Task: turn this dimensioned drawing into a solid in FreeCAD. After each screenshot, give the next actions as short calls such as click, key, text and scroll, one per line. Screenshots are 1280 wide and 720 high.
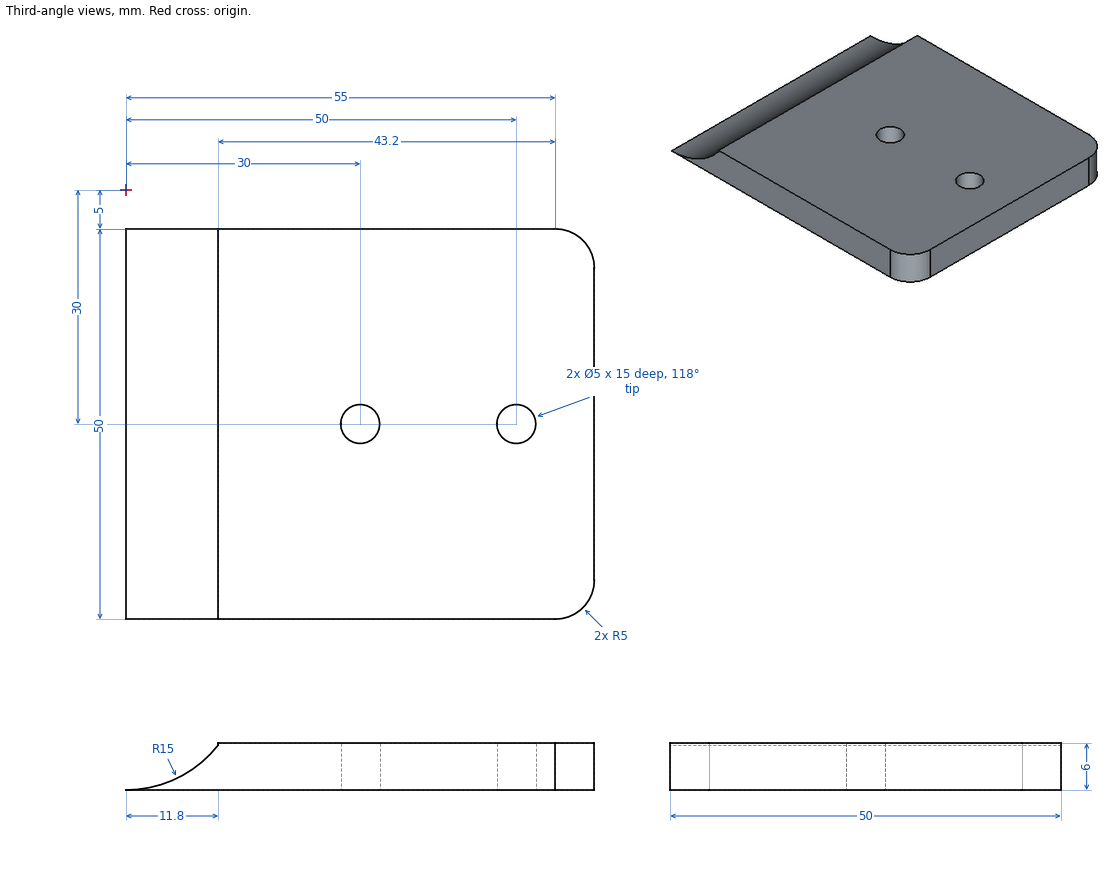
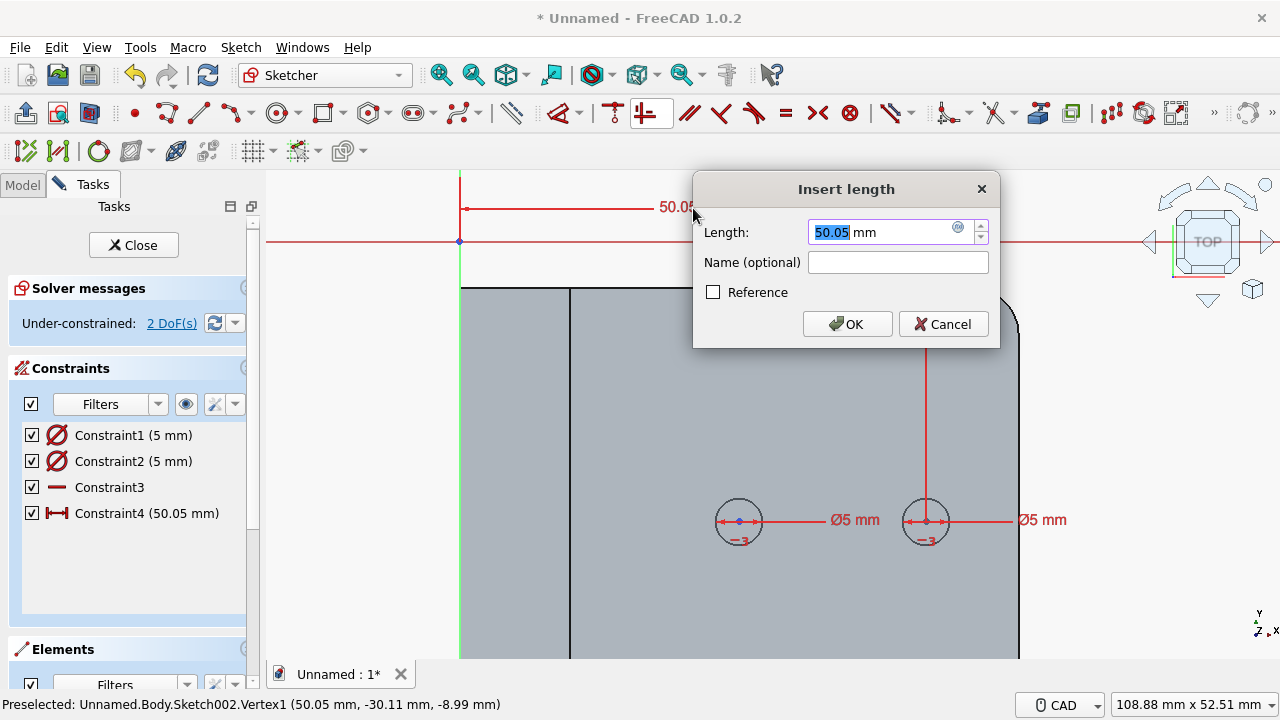
text(50)
key(Return)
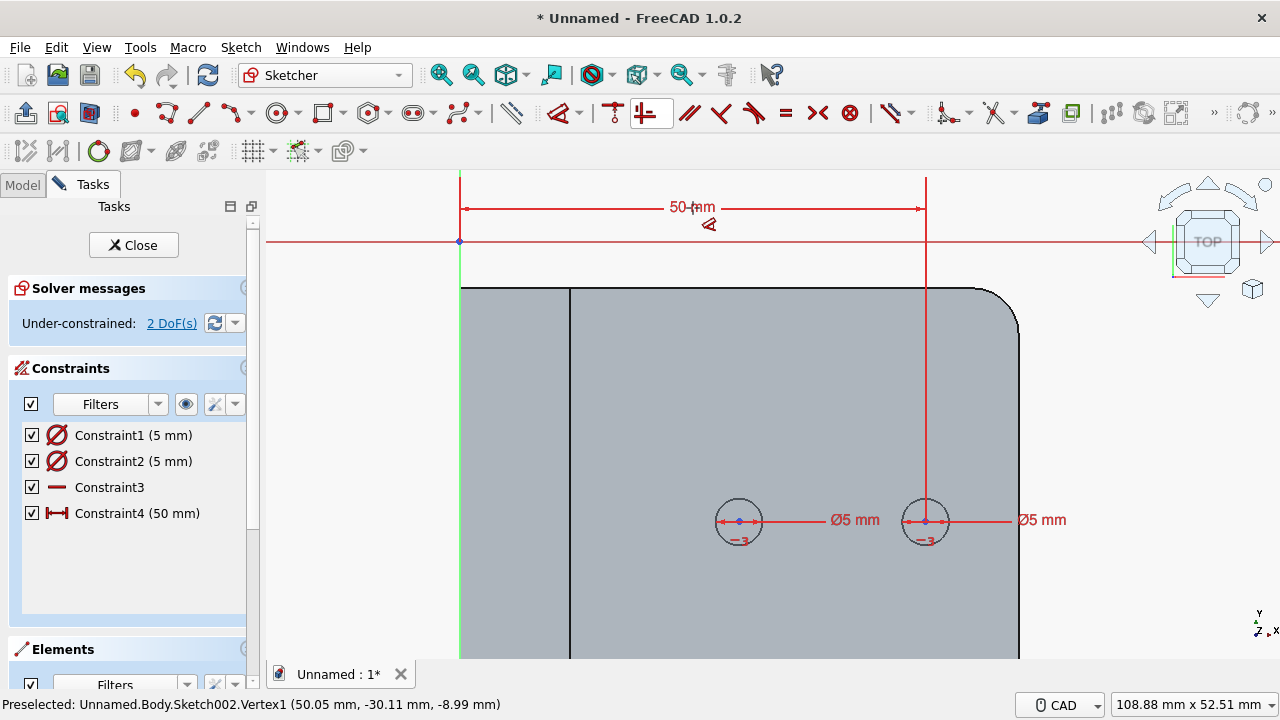
click(926, 522)
click(426, 382)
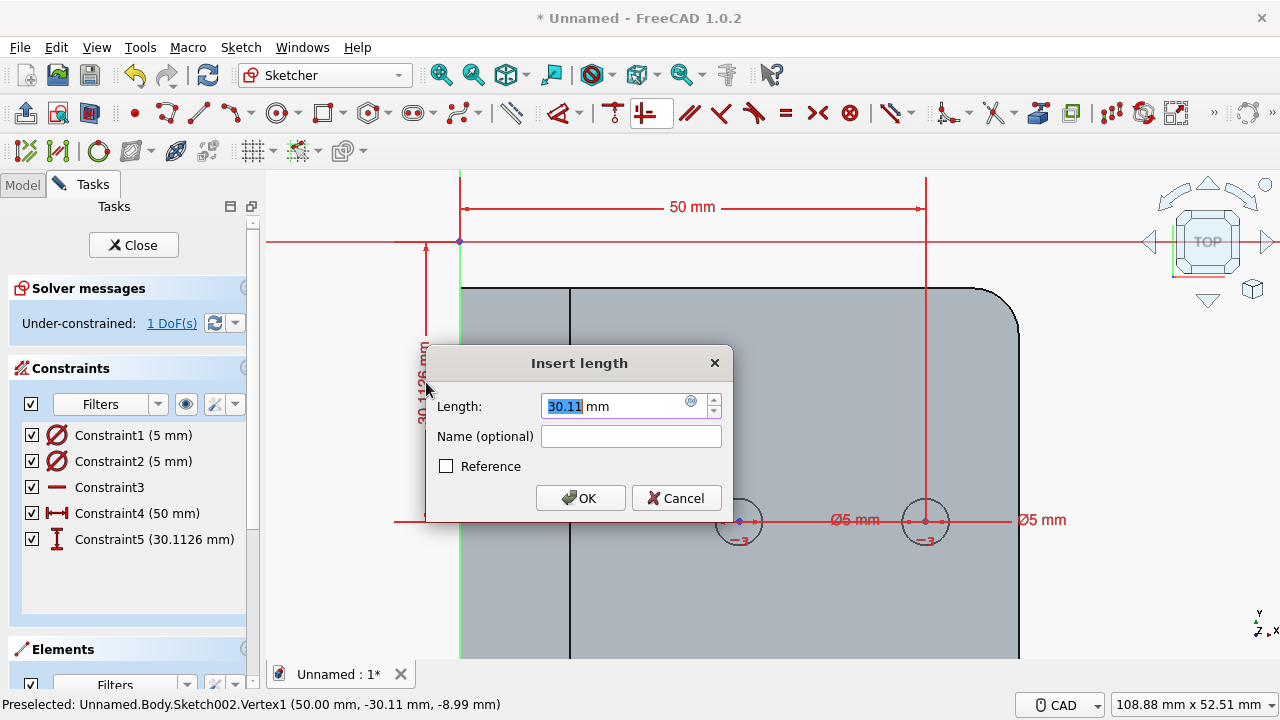
text(30)
key(Return)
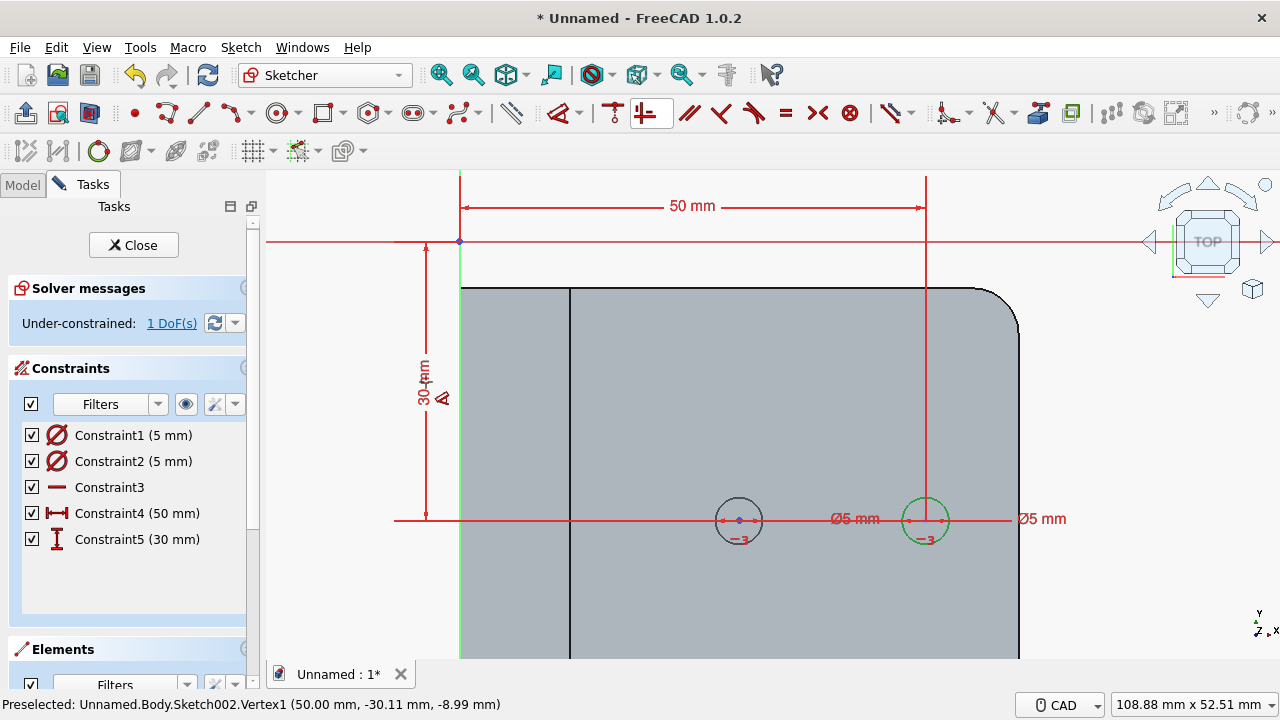
click(739, 521)
click(599, 208)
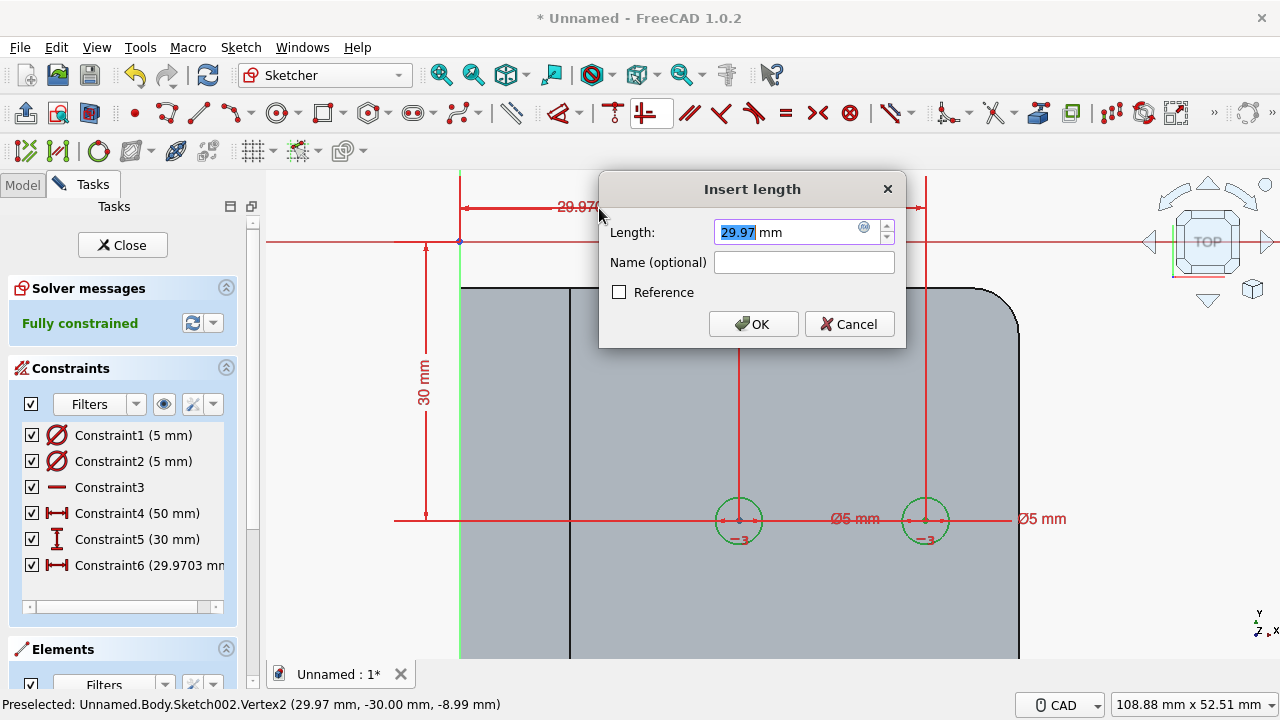
text(30)
key(Return)
key(Escape)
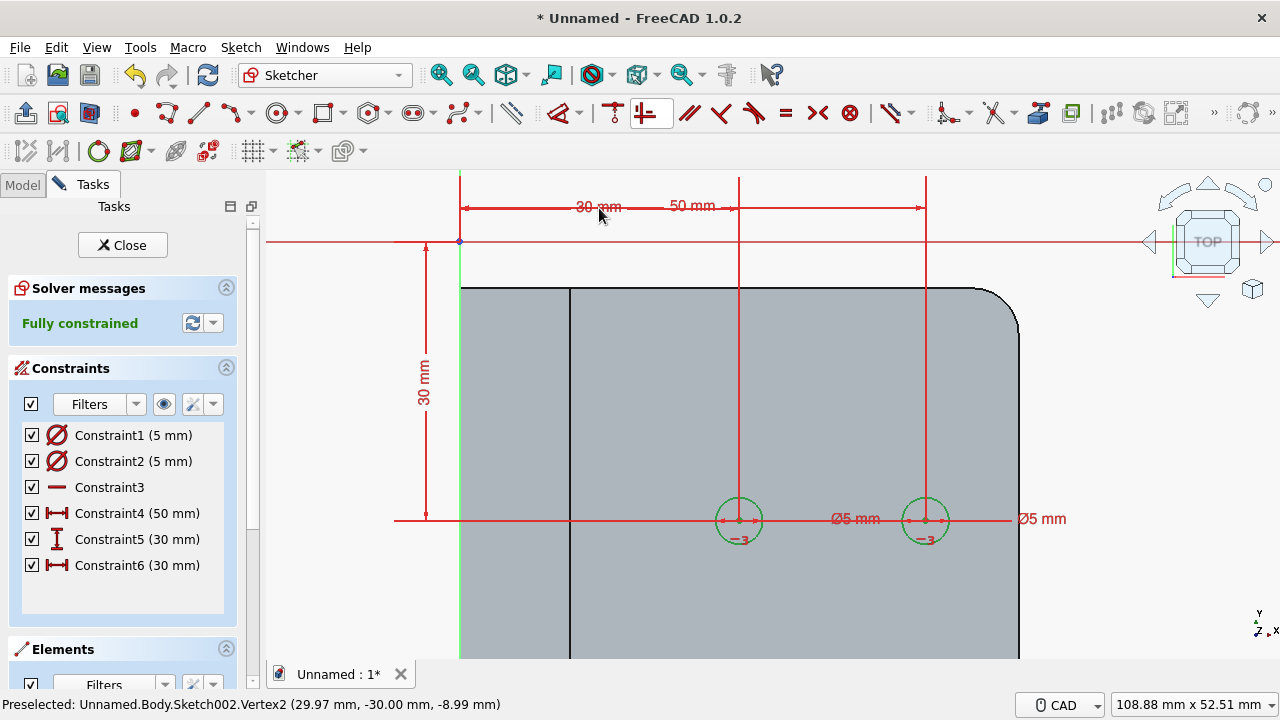
click(123, 245)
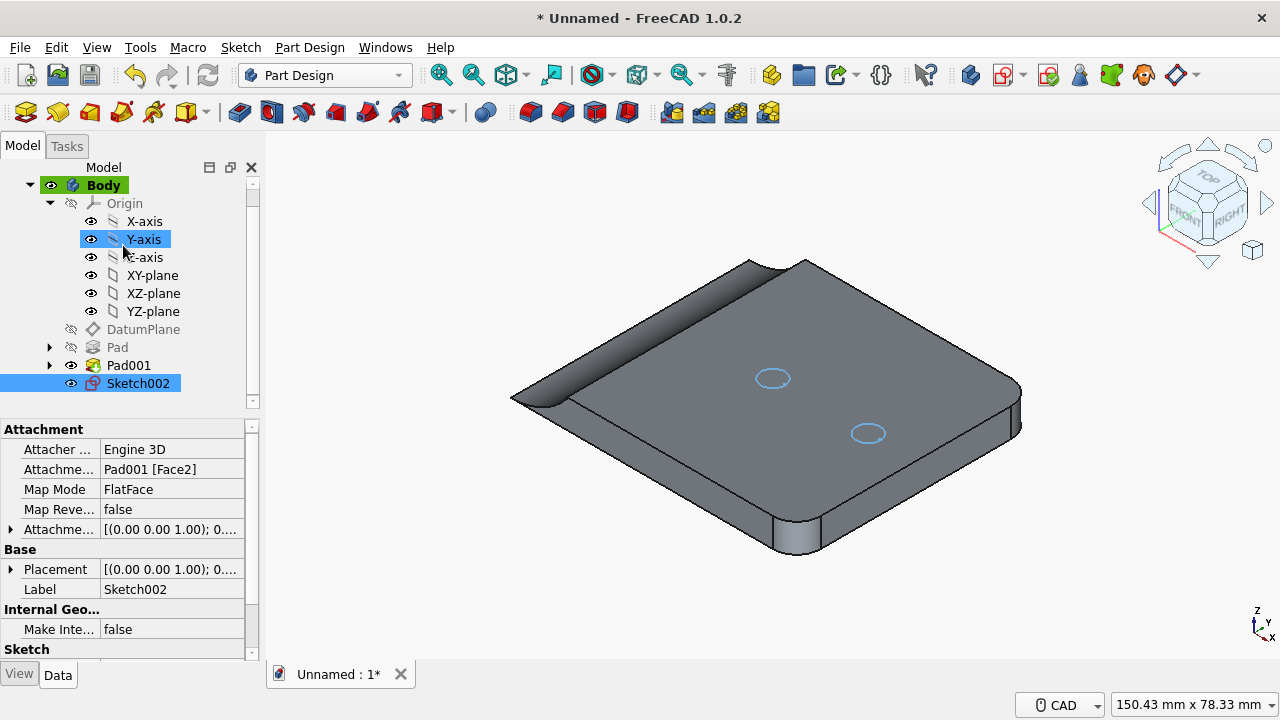
click(272, 112)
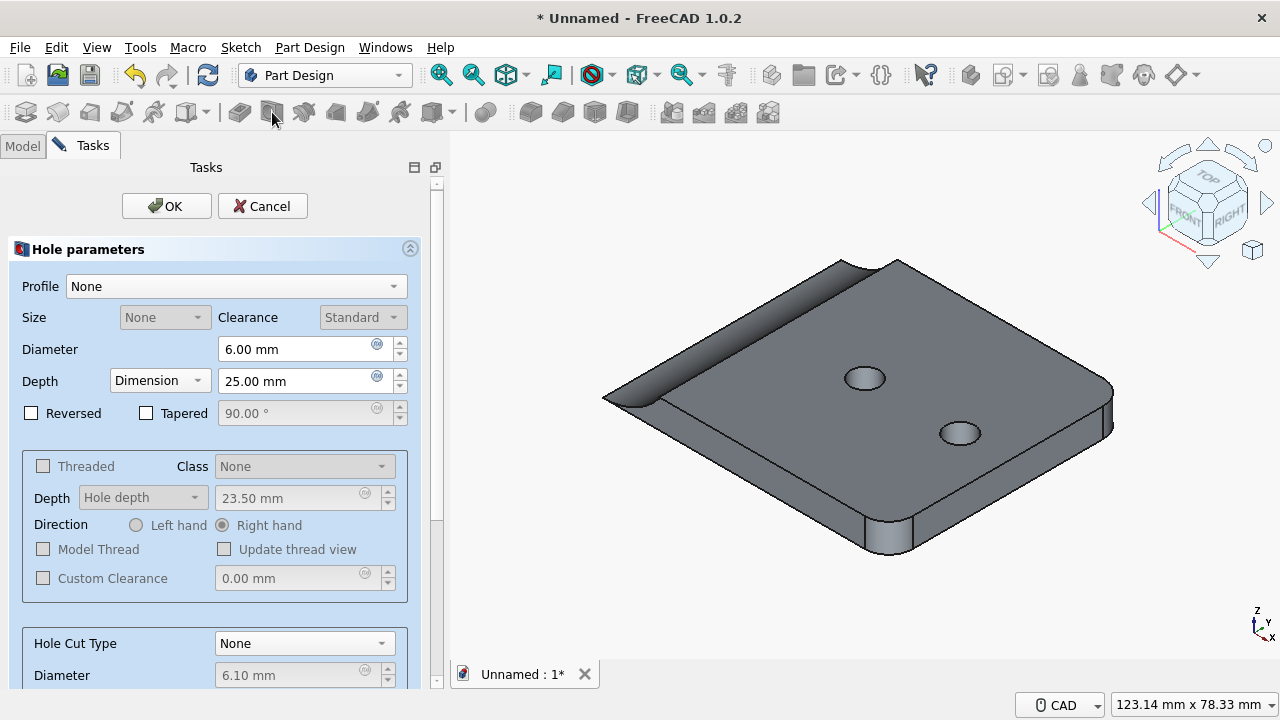
triple_click(305, 349)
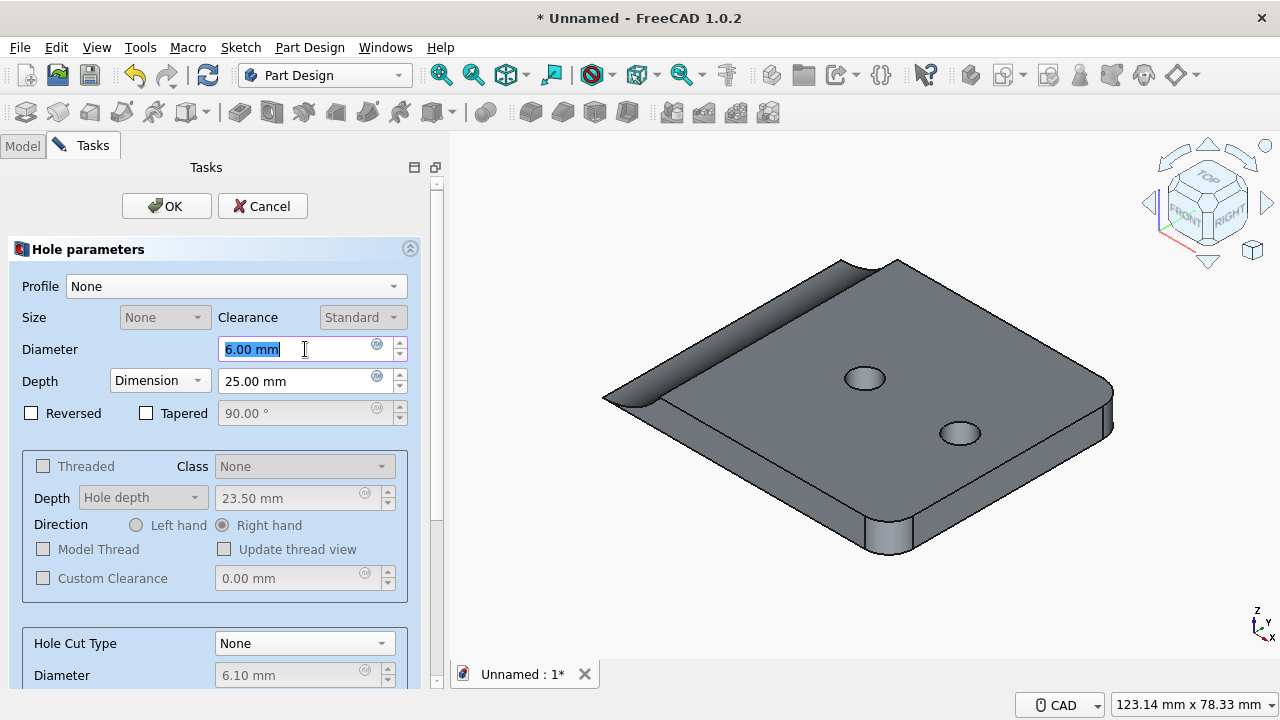
text(5)
key(Tab)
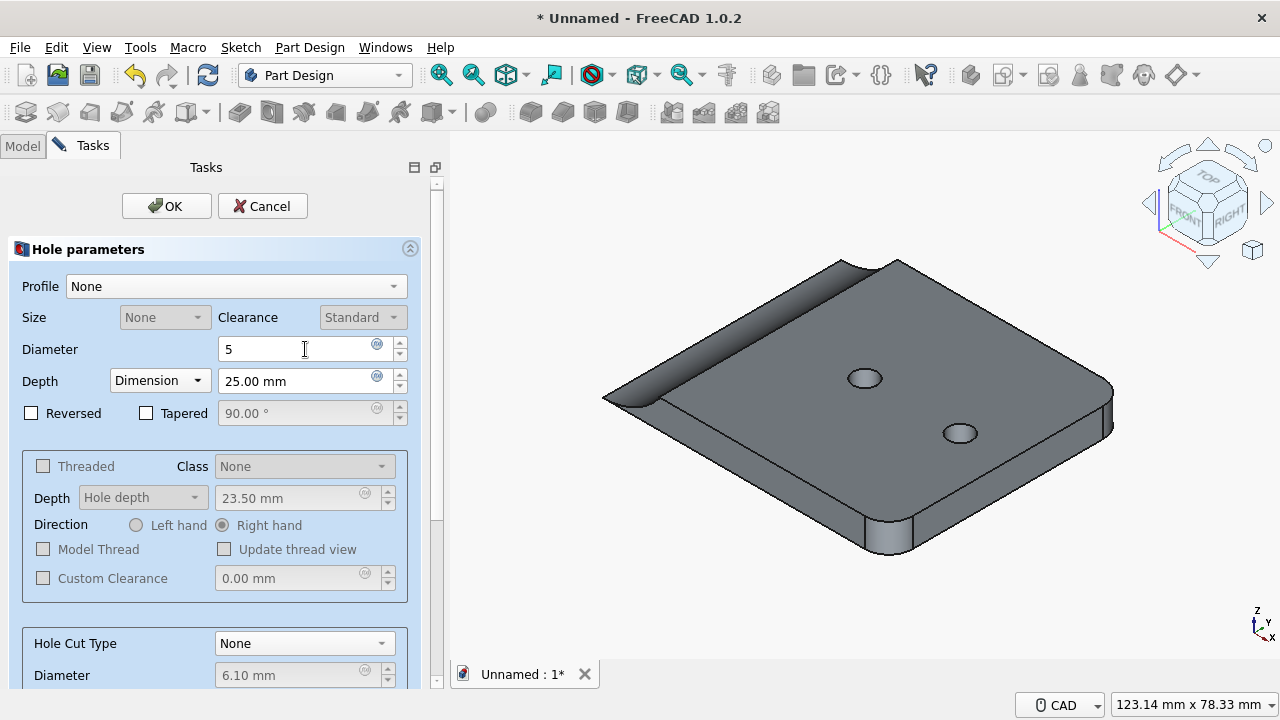
triple_click(305, 381)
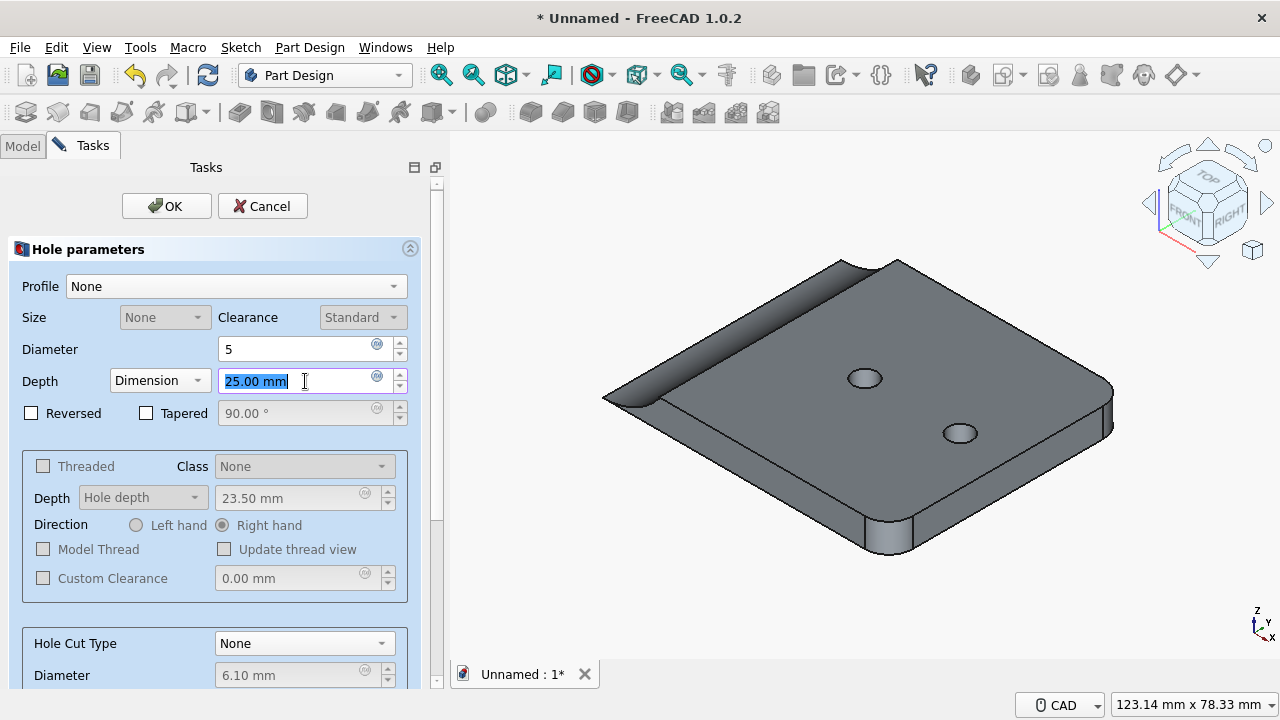
text(15)
key(Tab)